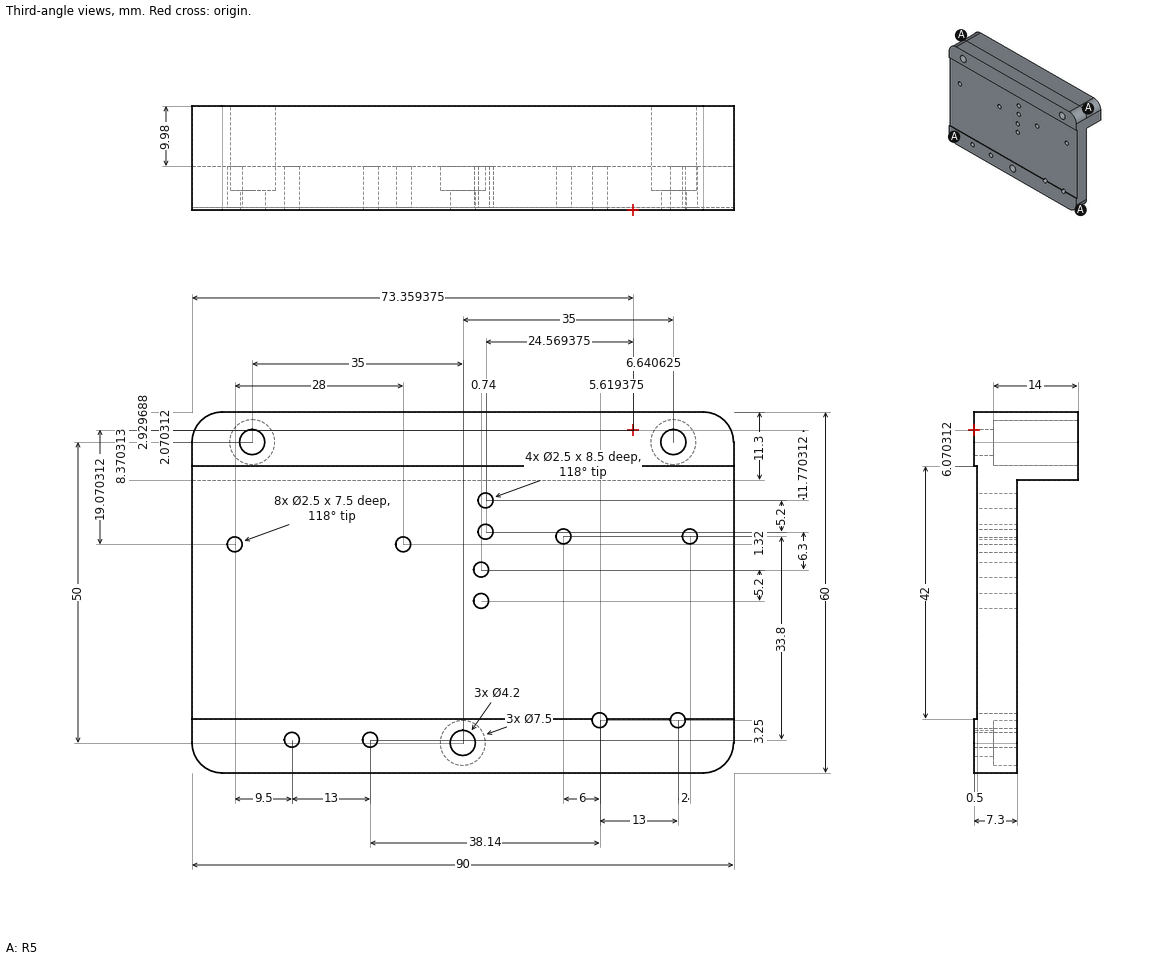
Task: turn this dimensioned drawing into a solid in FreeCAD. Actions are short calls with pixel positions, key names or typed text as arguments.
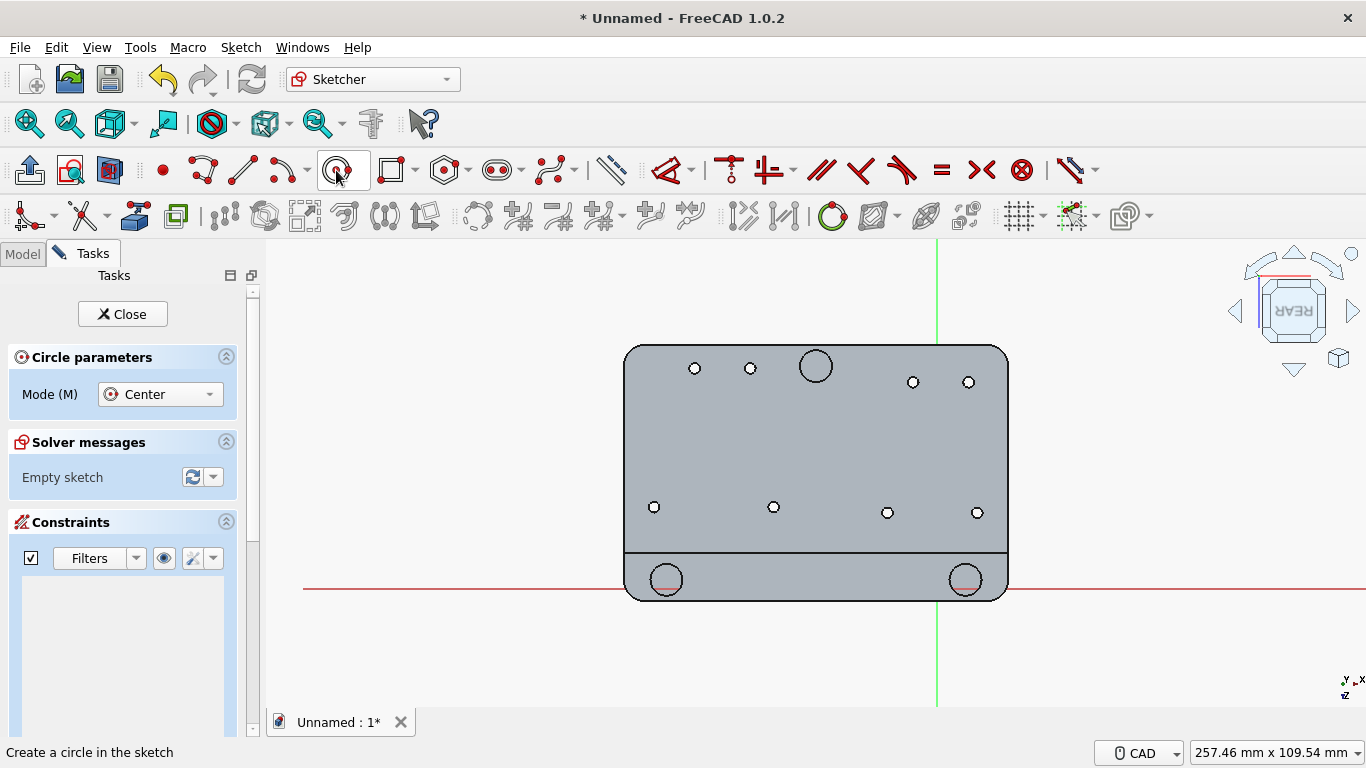
scroll(816, 366, up, 5)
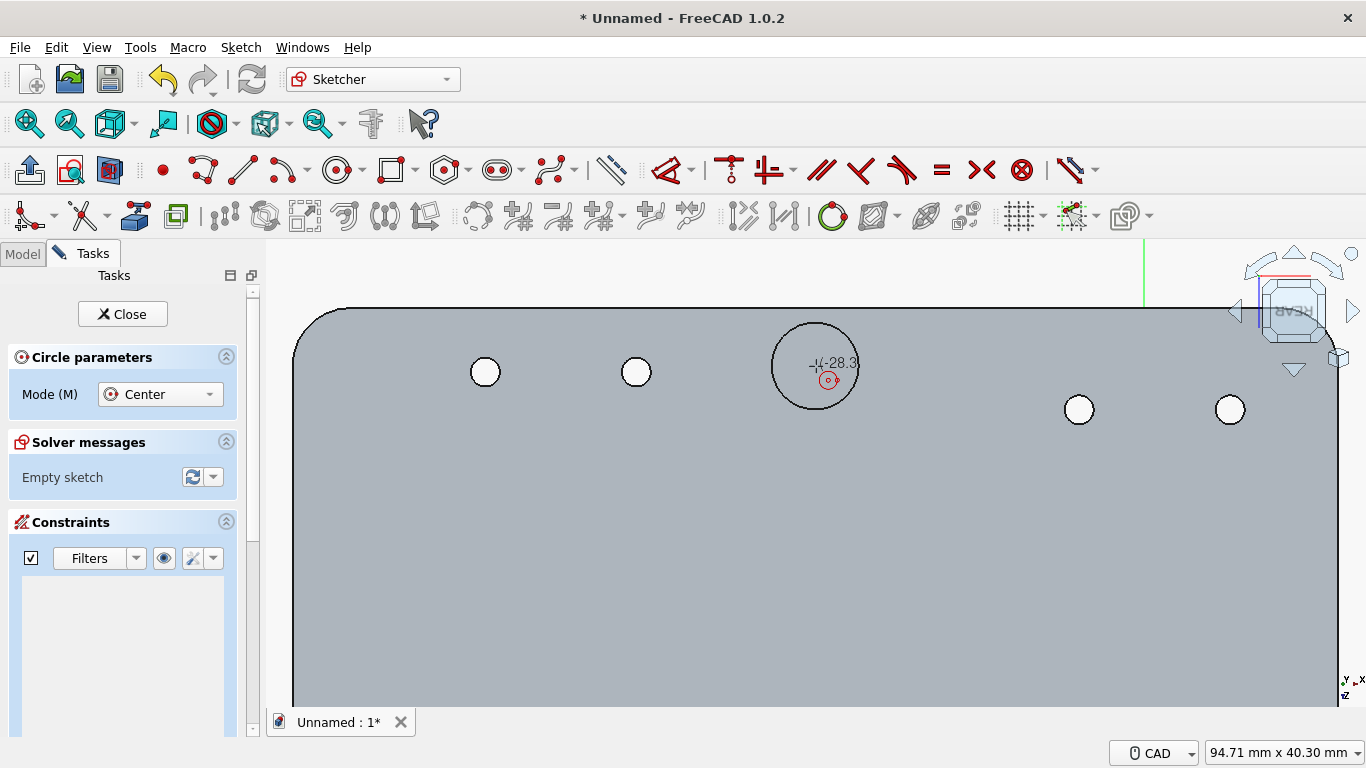
click(815, 366)
move(832, 349)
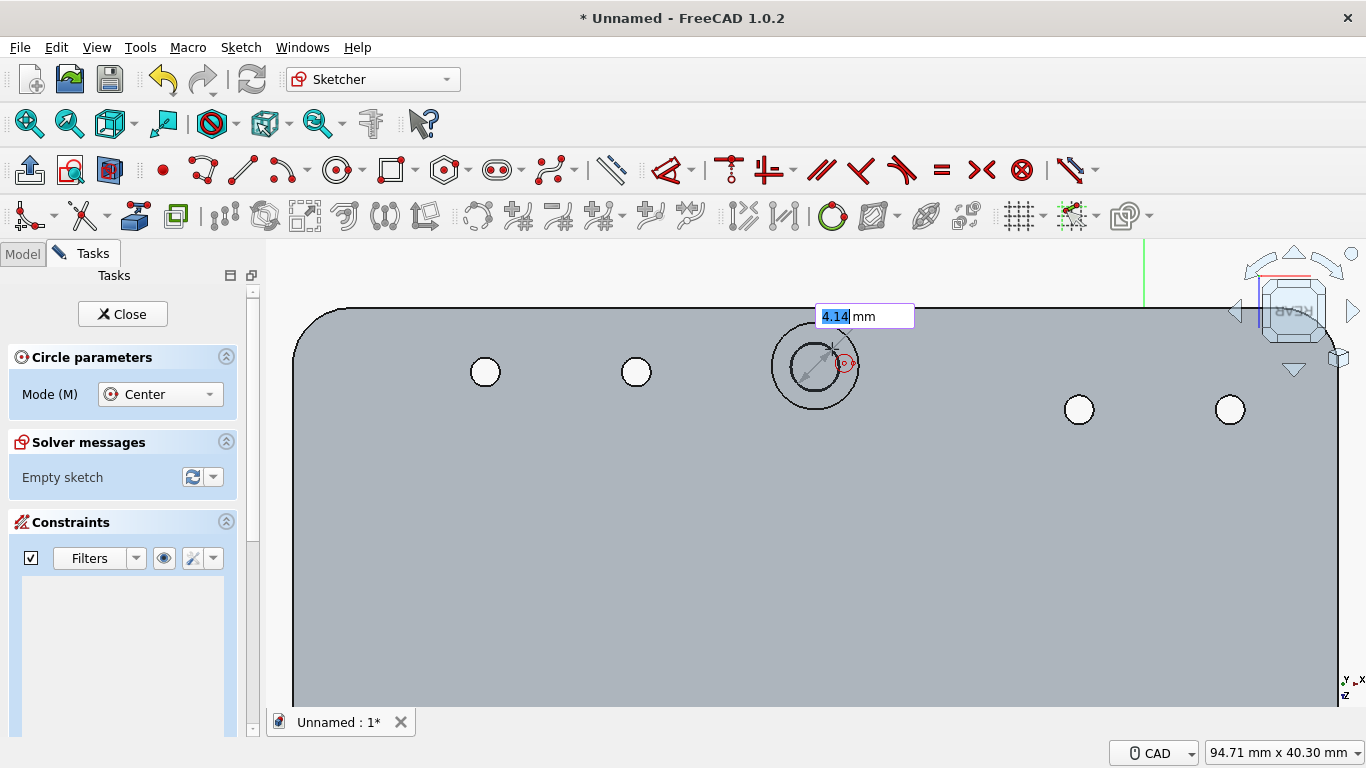
text(4.2)
key(Return)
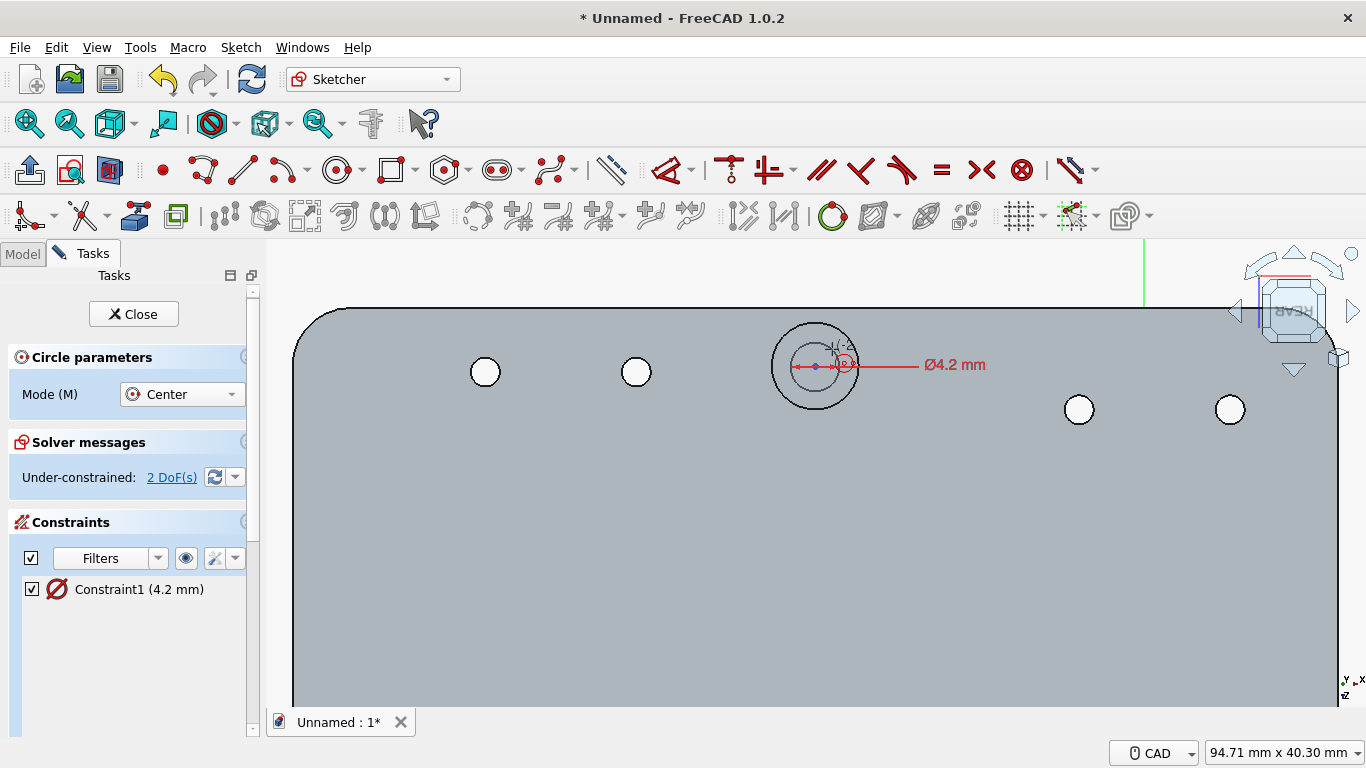
scroll(692, 323, down, 4)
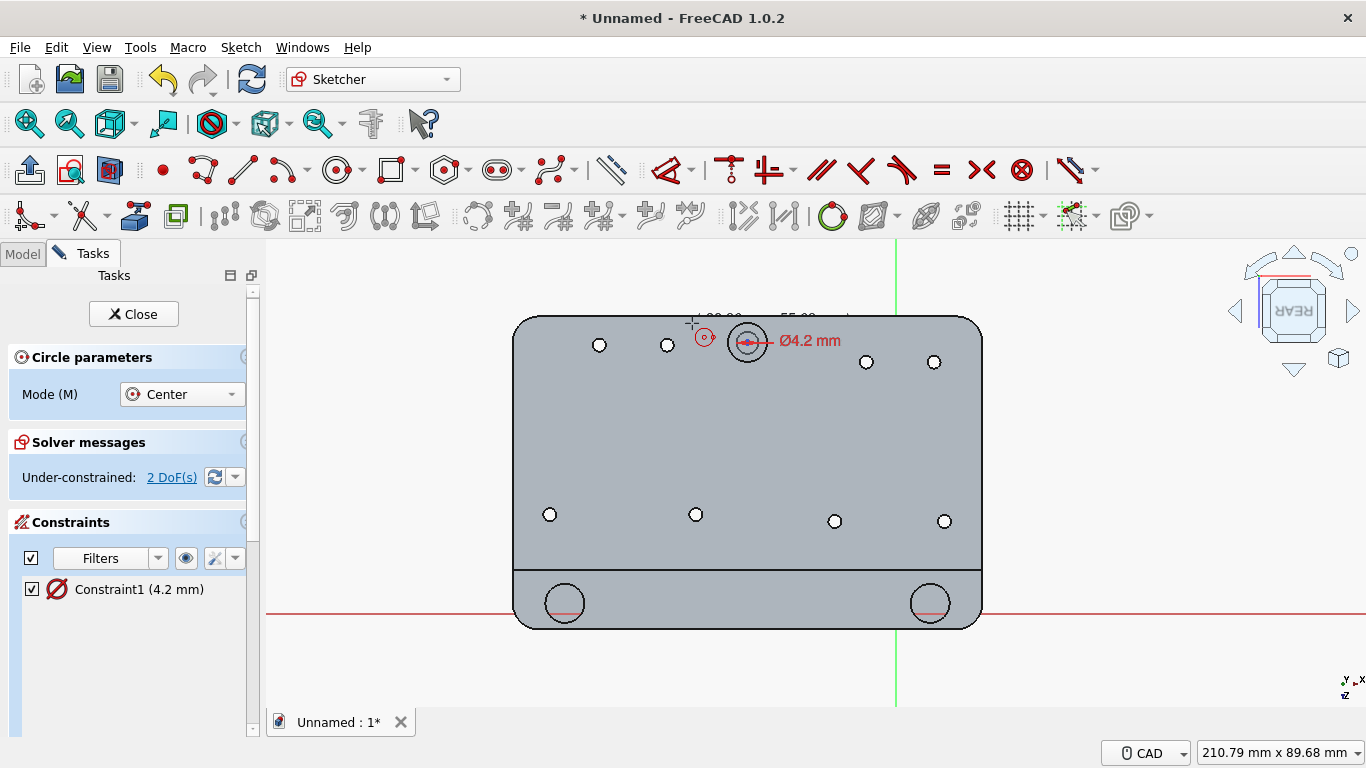
scroll(565, 603, up, 4)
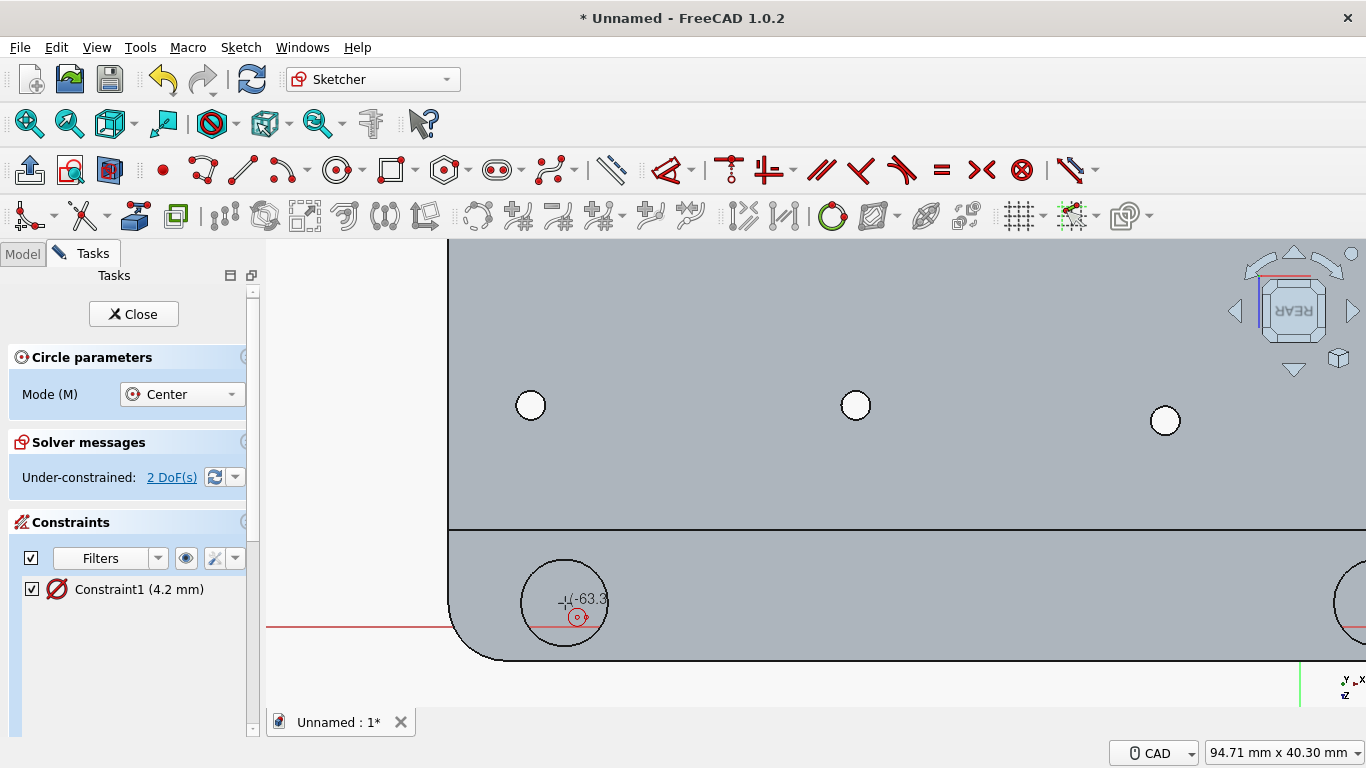
click(564, 603)
move(582, 586)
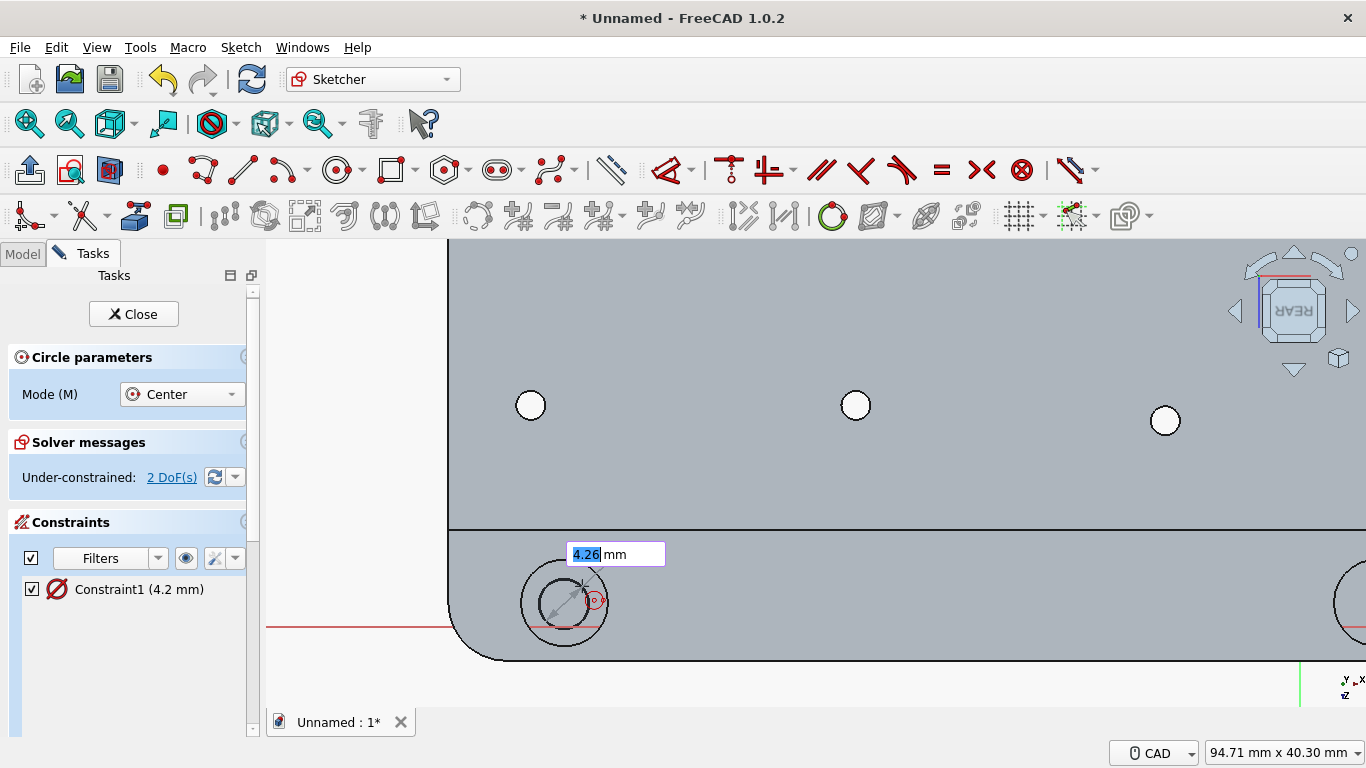
text(4.2)
key(Return)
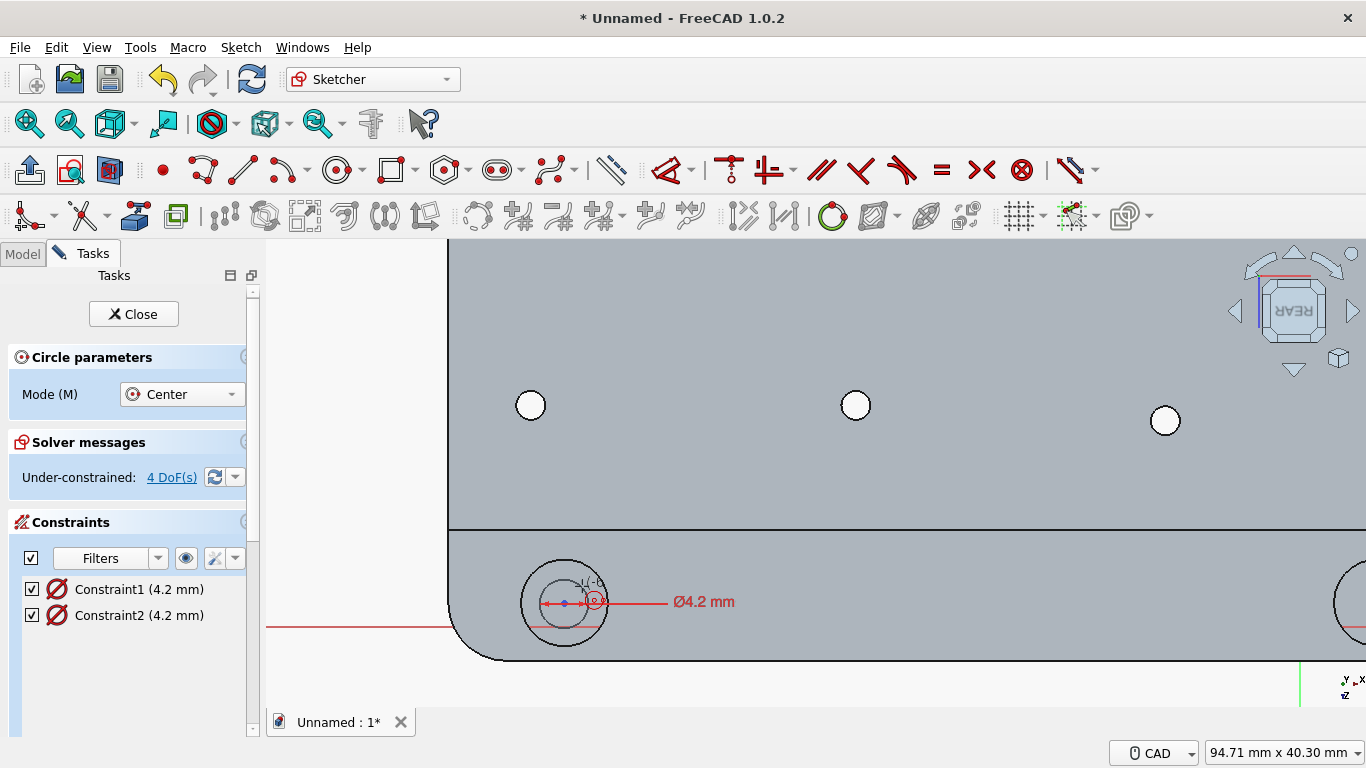
scroll(565, 604, down, 4)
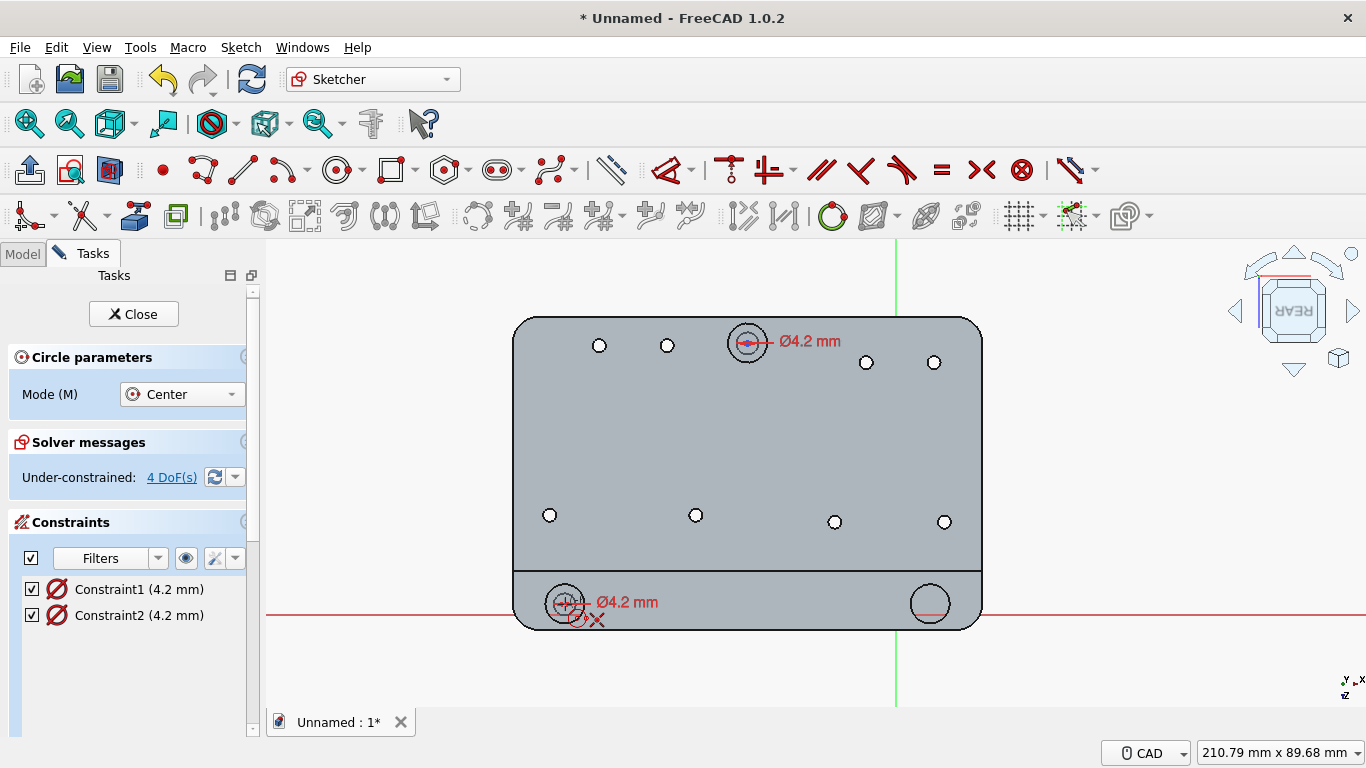
scroll(930, 604, up, 4)